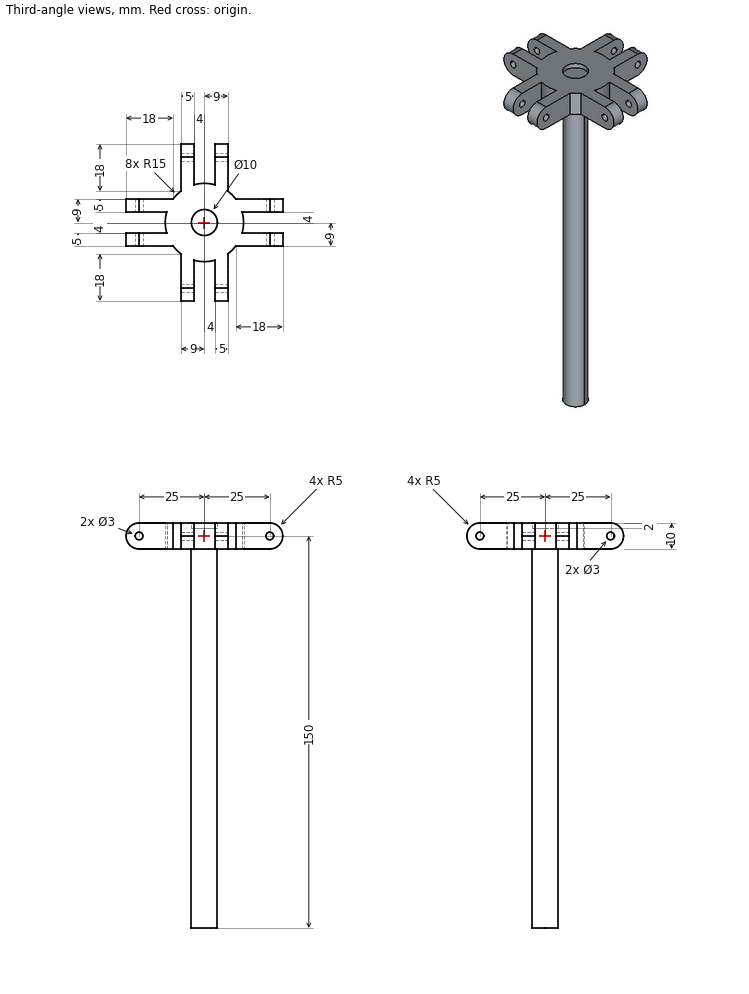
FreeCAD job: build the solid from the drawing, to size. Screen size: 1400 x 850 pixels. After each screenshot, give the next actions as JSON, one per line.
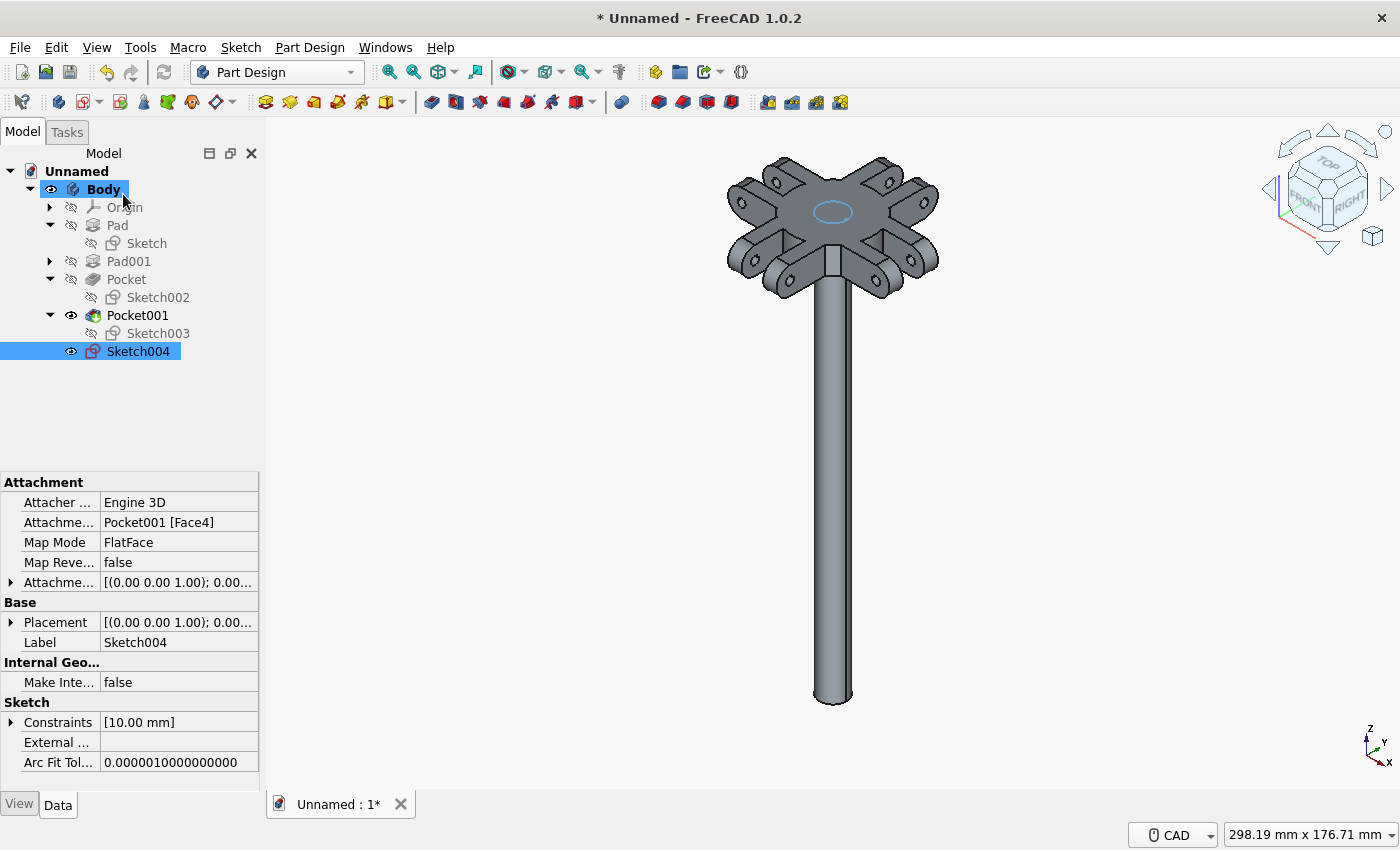
{"action": "left_click", "coordinate": [432, 102]}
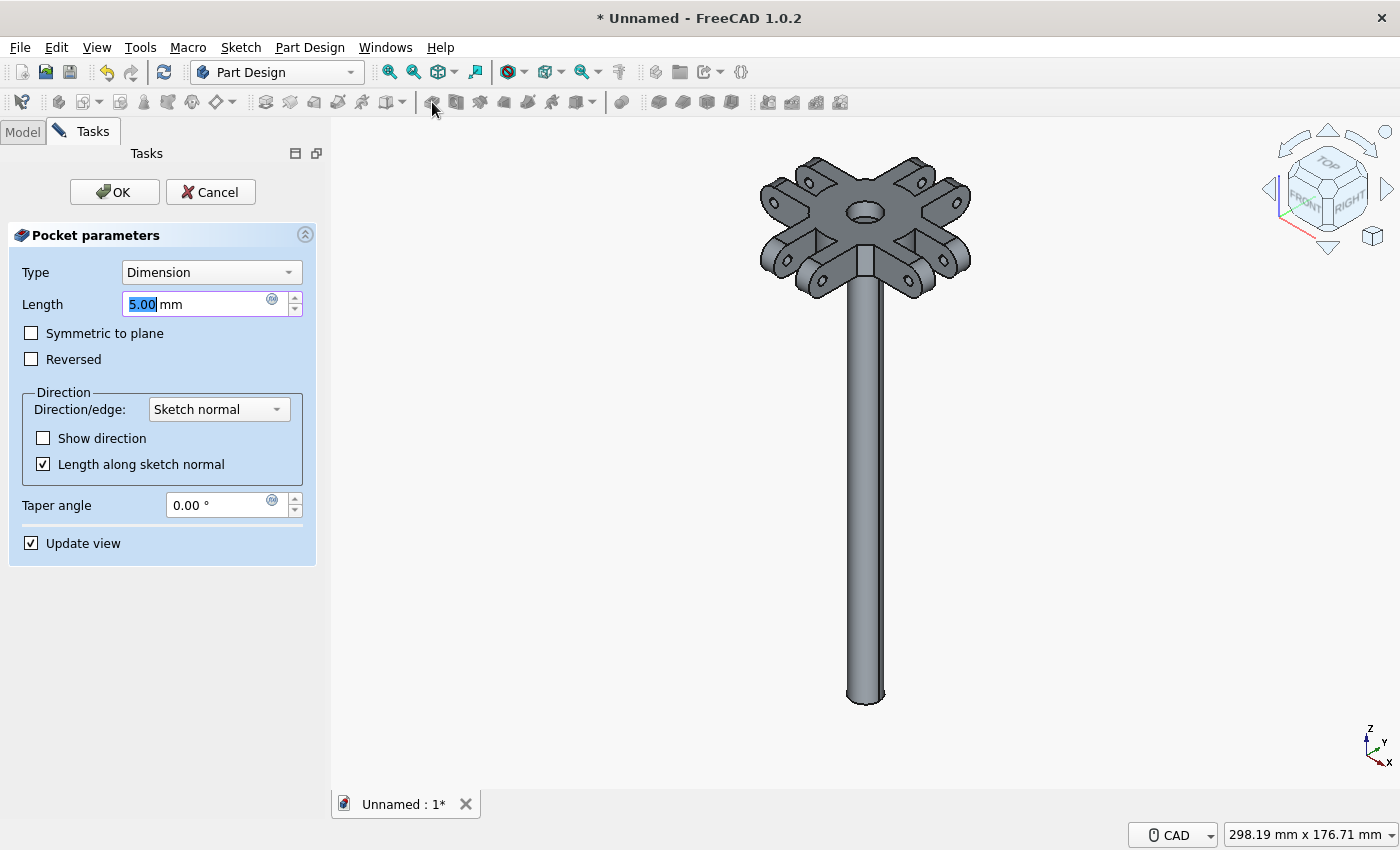
{"action": "type", "text": "2"}
{"action": "key", "text": "Tab"}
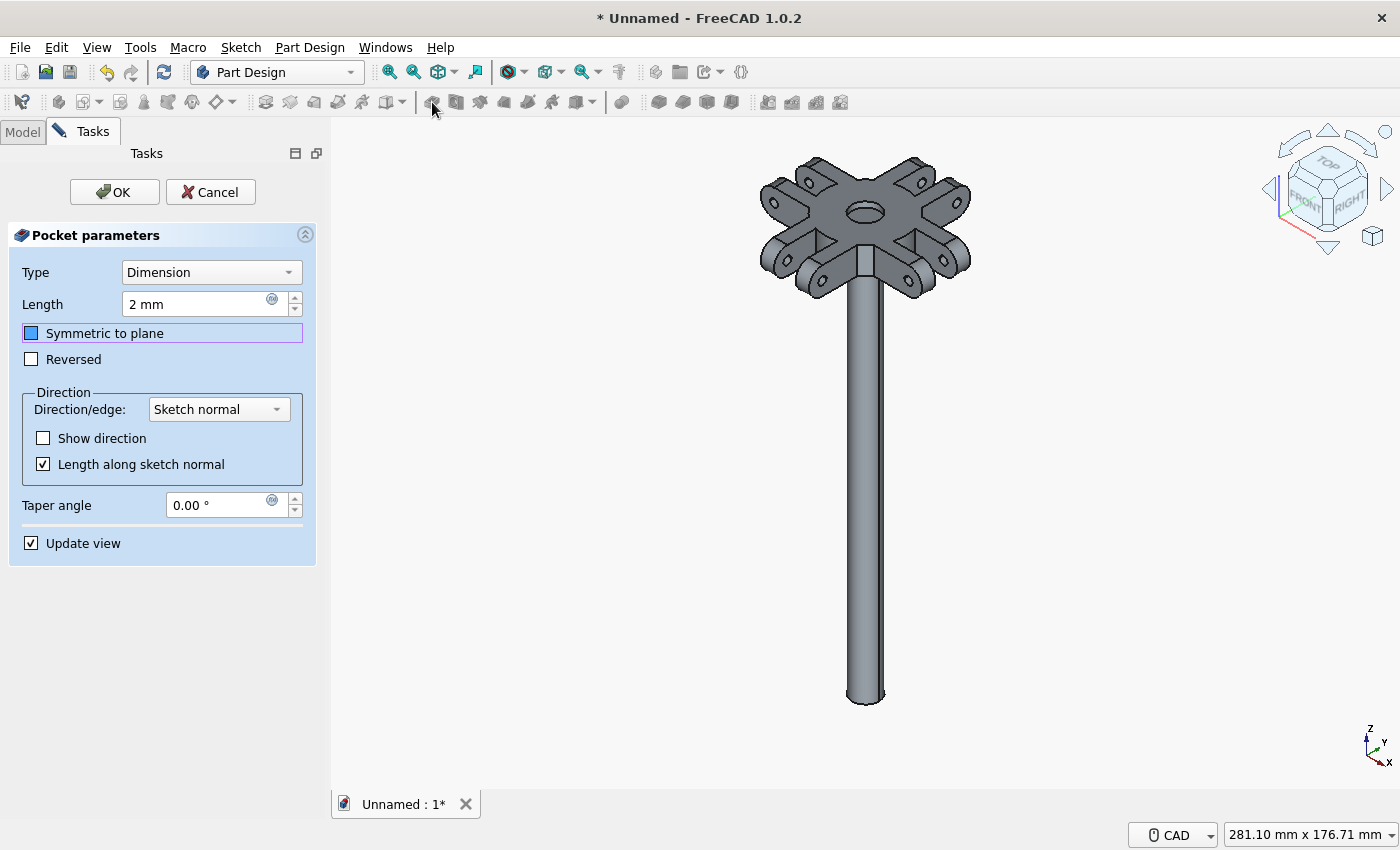
{"action": "left_click", "coordinate": [115, 192]}